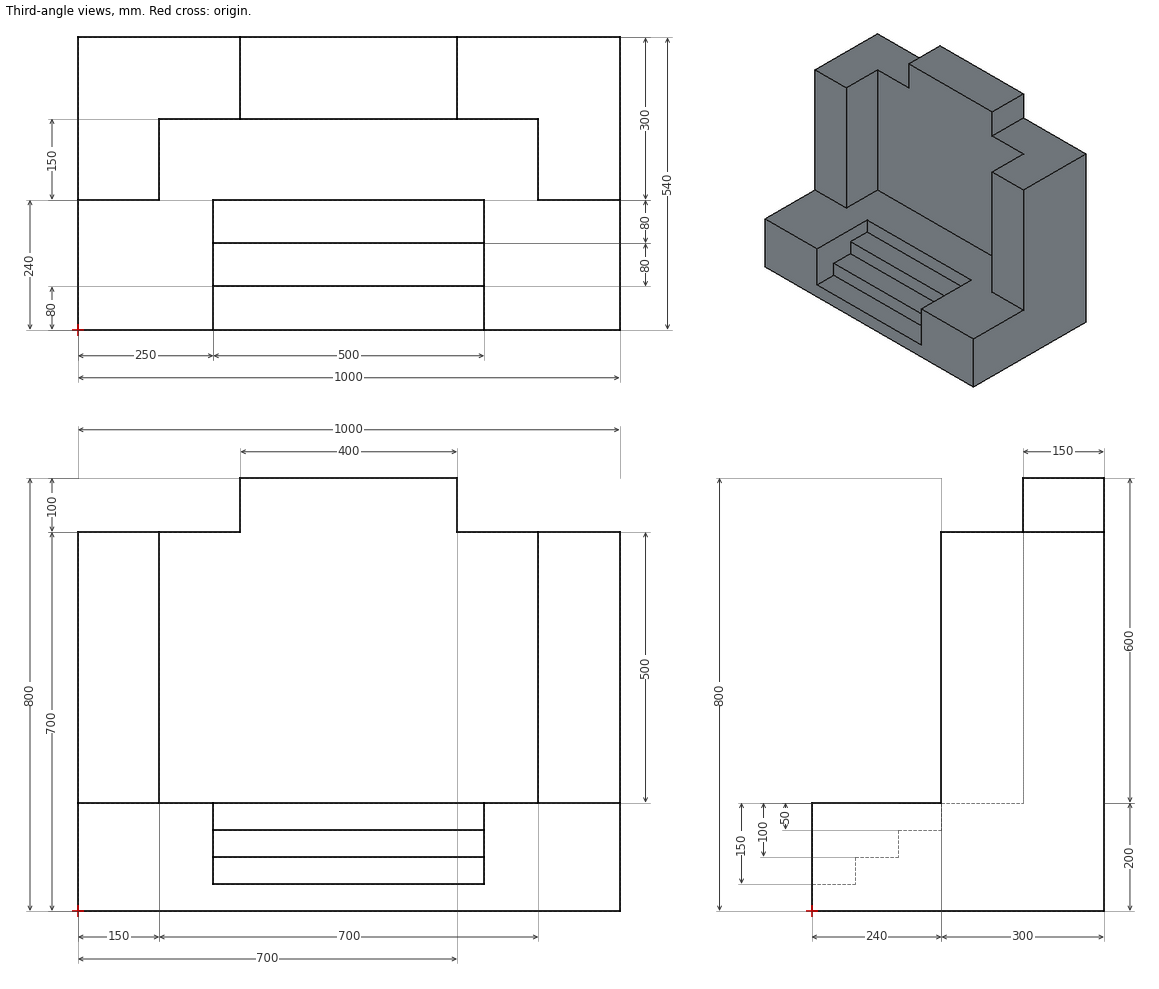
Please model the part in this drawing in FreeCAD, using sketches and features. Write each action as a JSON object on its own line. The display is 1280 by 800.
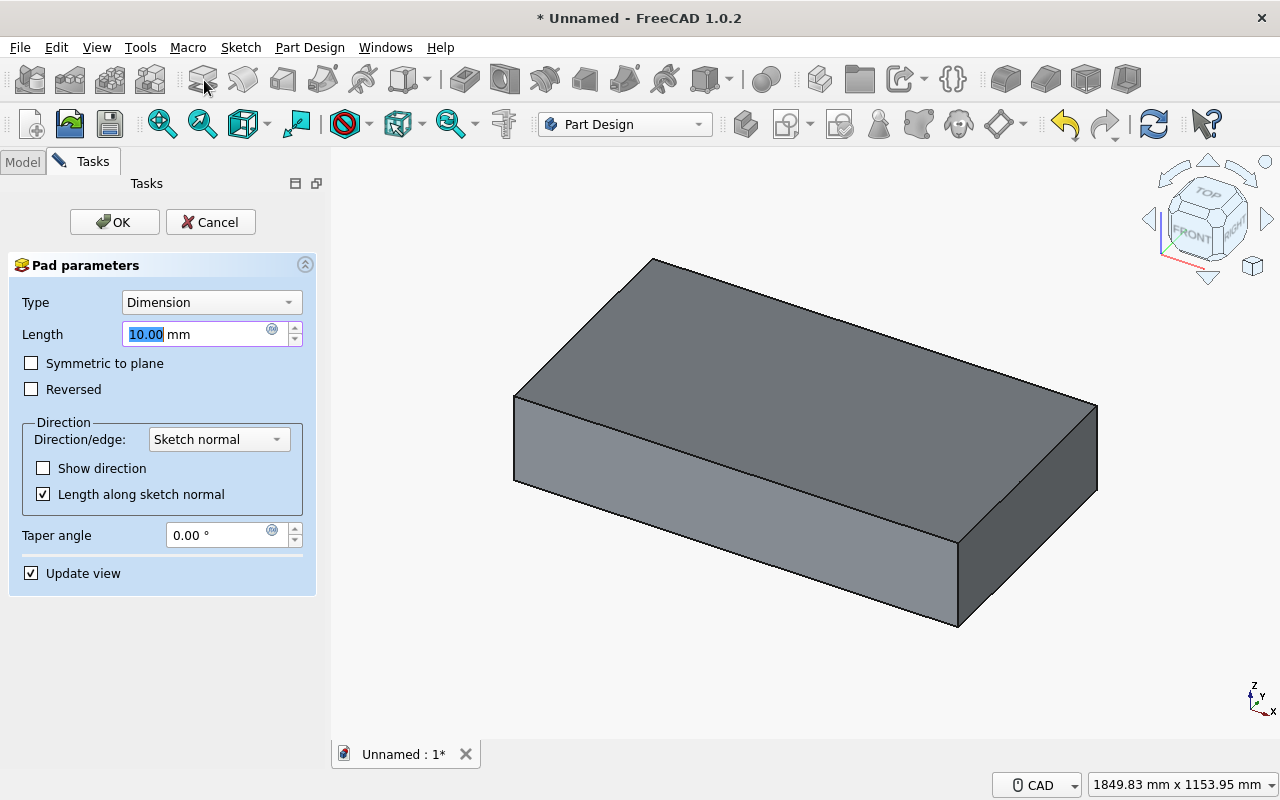
{"action": "type", "text": "1000"}
{"action": "key", "text": "Tab"}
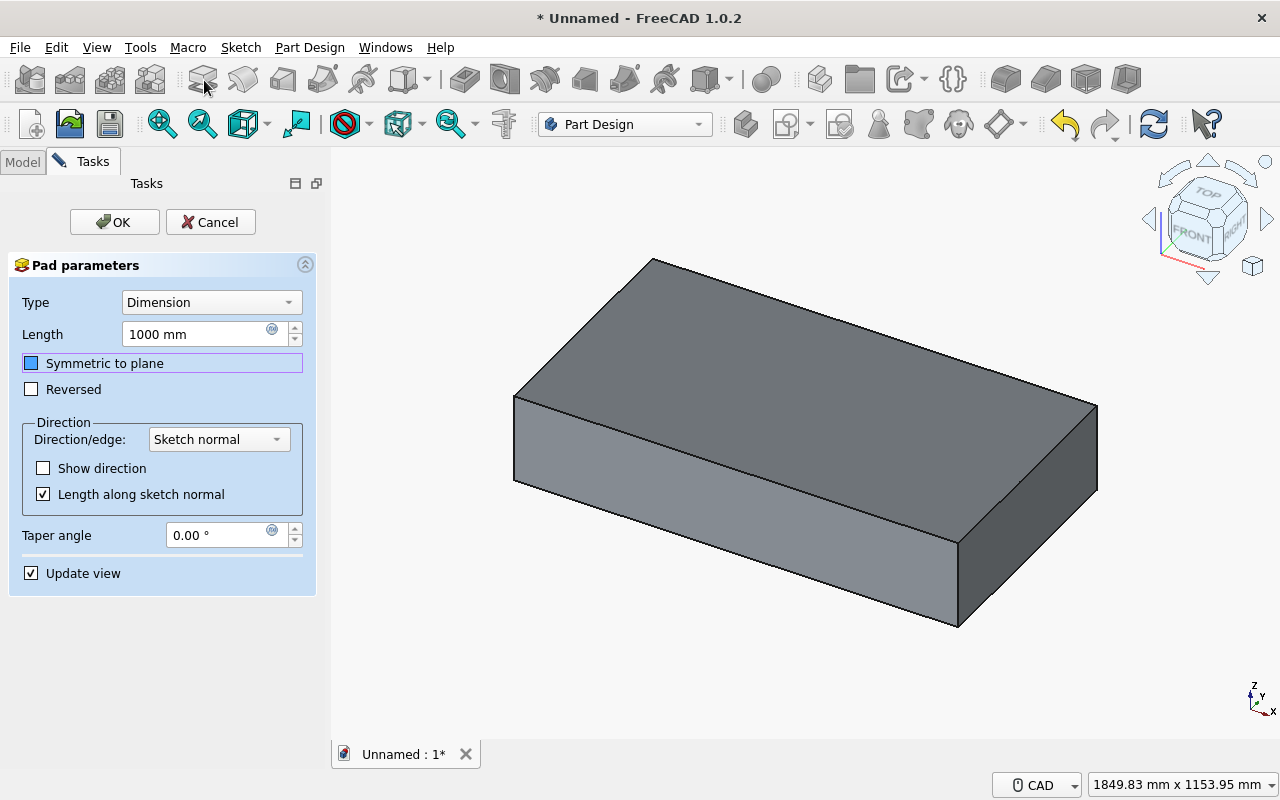
{"action": "left_click", "coordinate": [30, 389]}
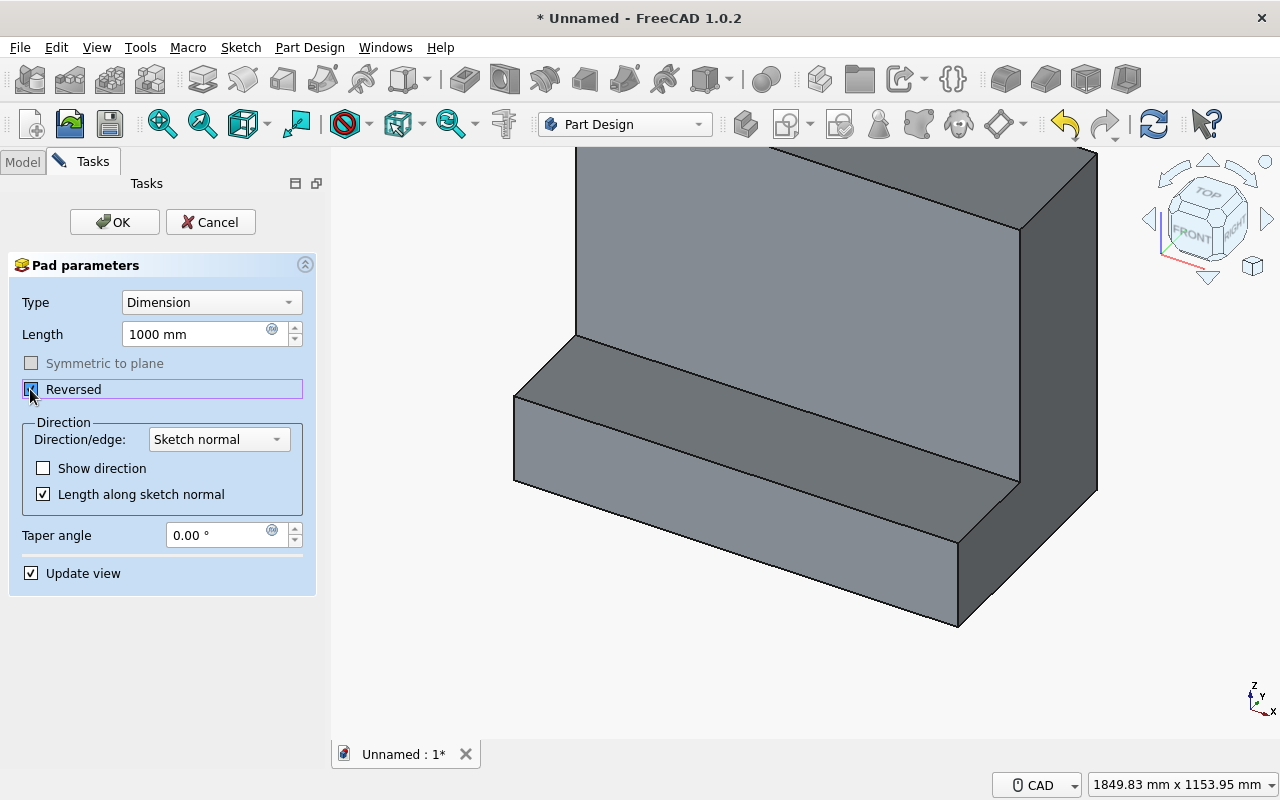
{"action": "left_click", "coordinate": [115, 222]}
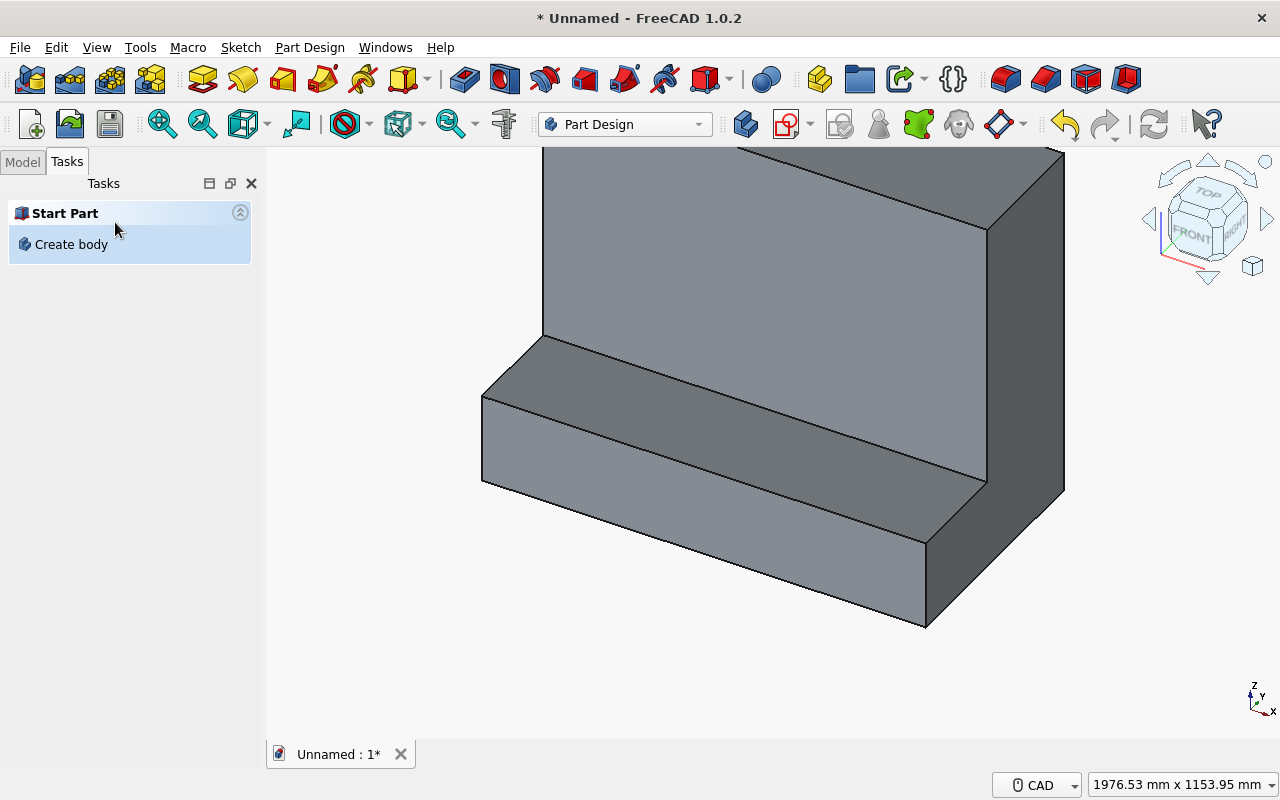
{"action": "left_click", "coordinate": [164, 124]}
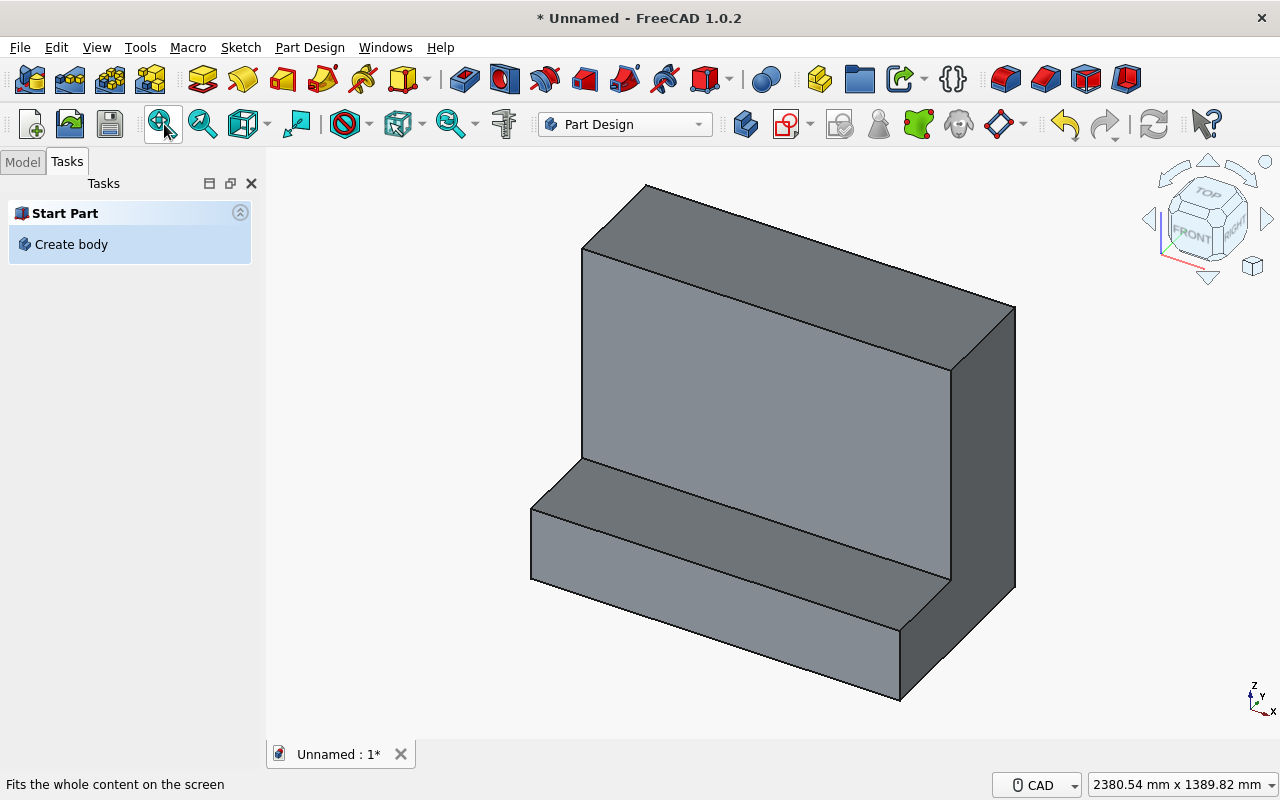
{"action": "left_click", "coordinate": [904, 312]}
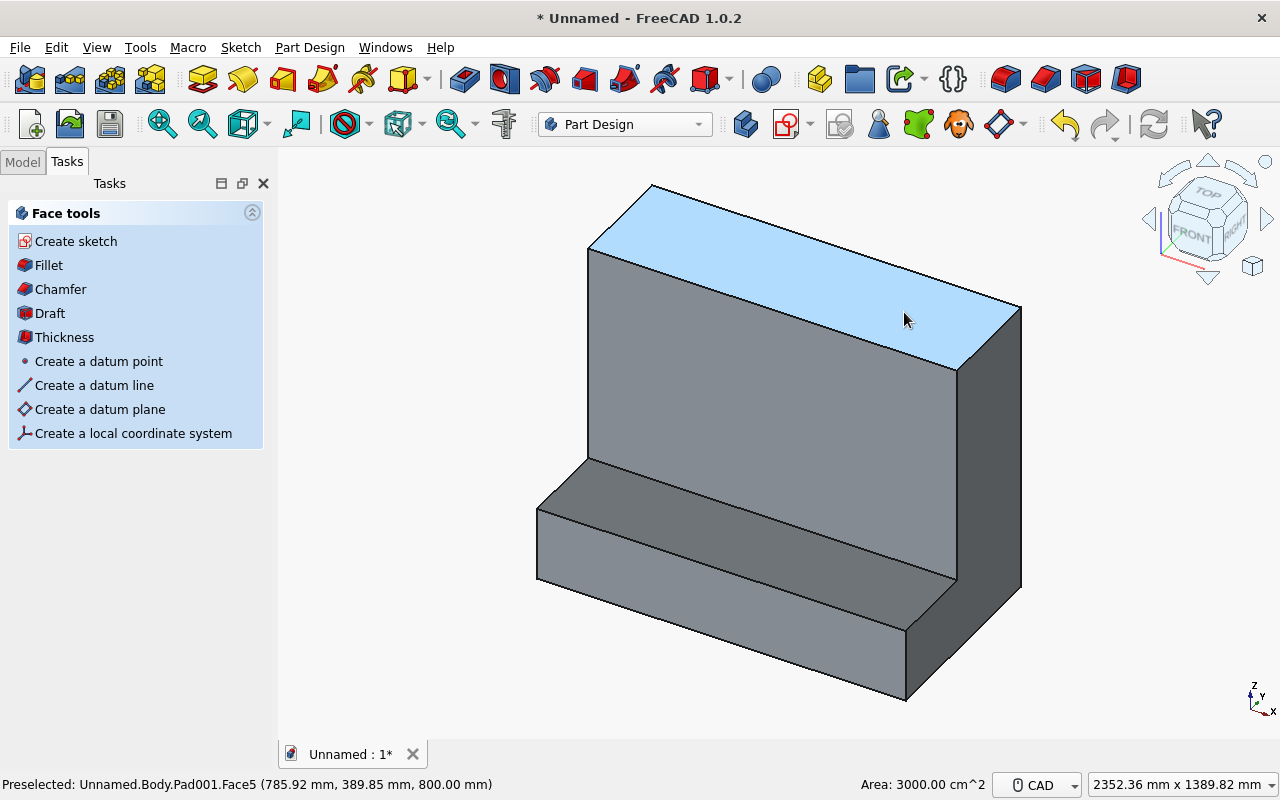
{"action": "left_click", "coordinate": [786, 124]}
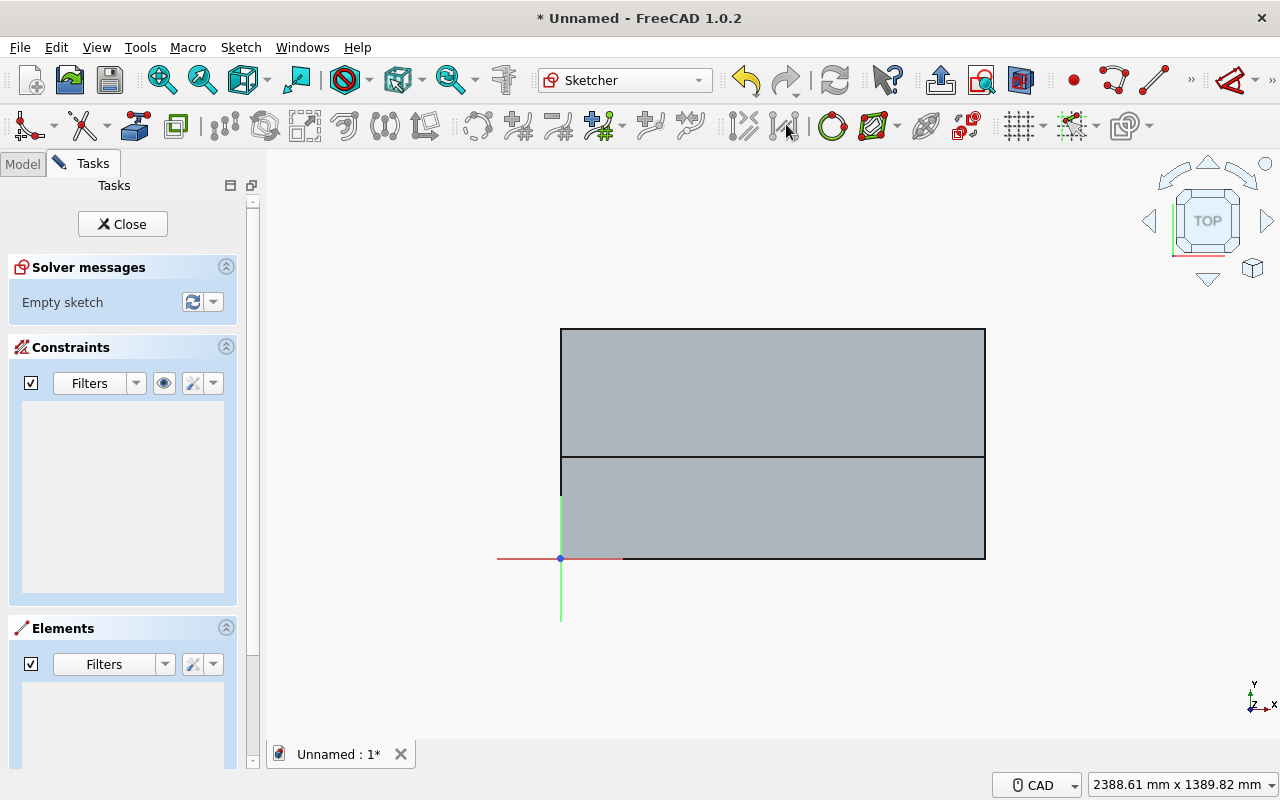
{"action": "scroll", "coordinate": [912, 444], "scroll_direction": "up", "scroll_amount": 2}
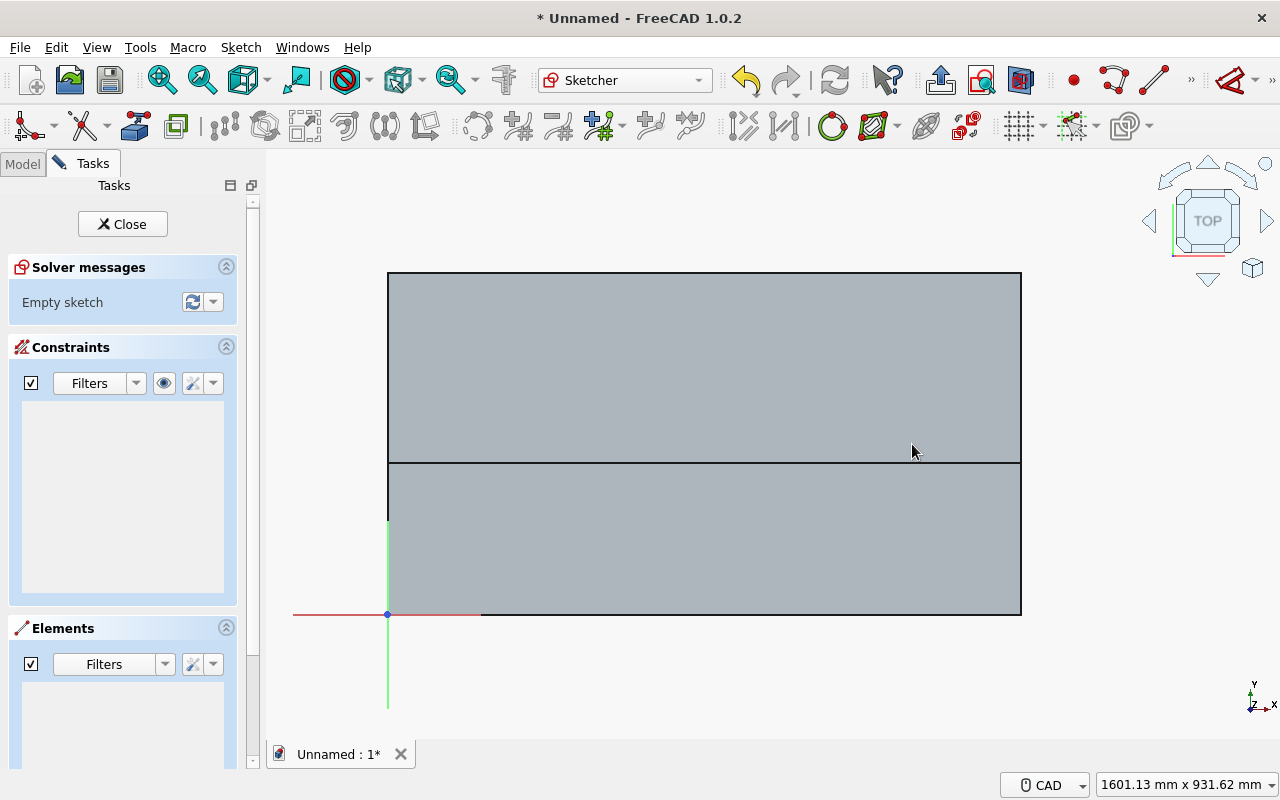
{"action": "key", "text": "g r"}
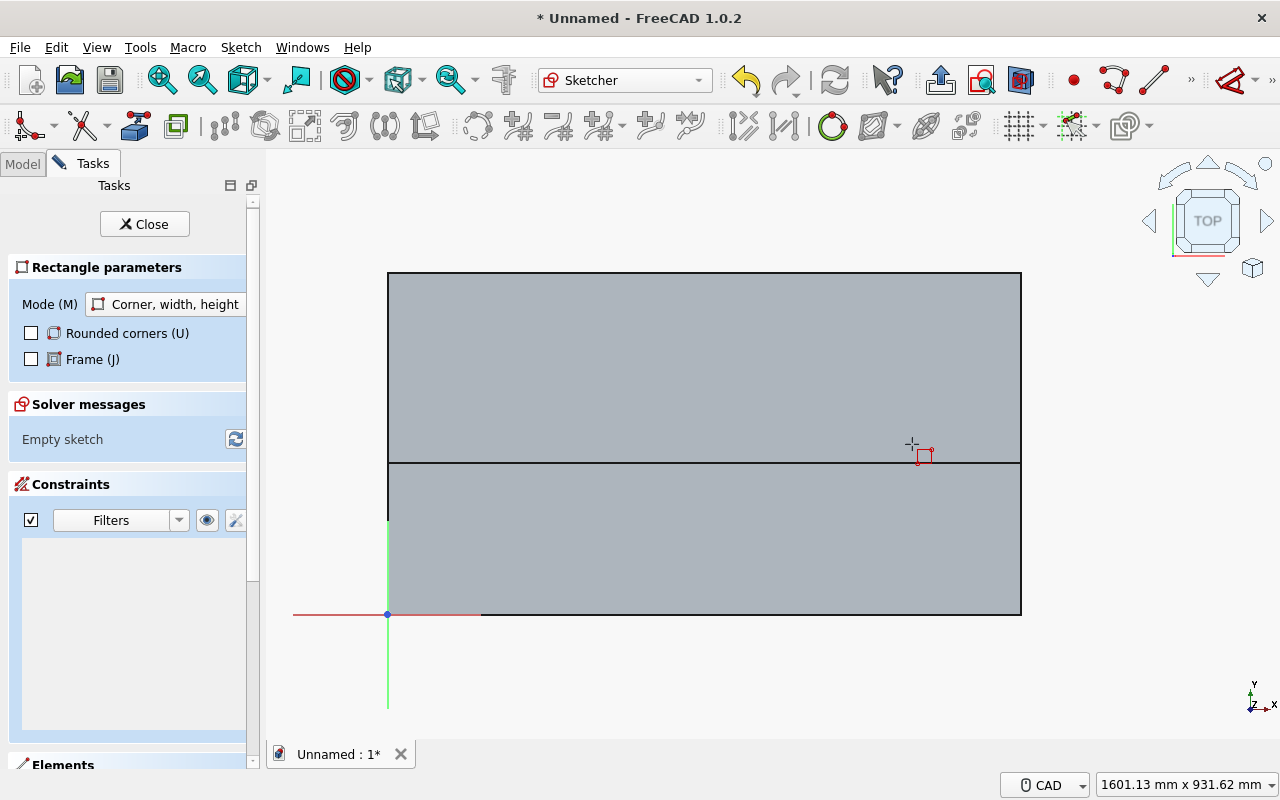
{"action": "left_click", "coordinate": [388, 273]}
{"action": "mouse_move", "coordinate": [1021, 463]}